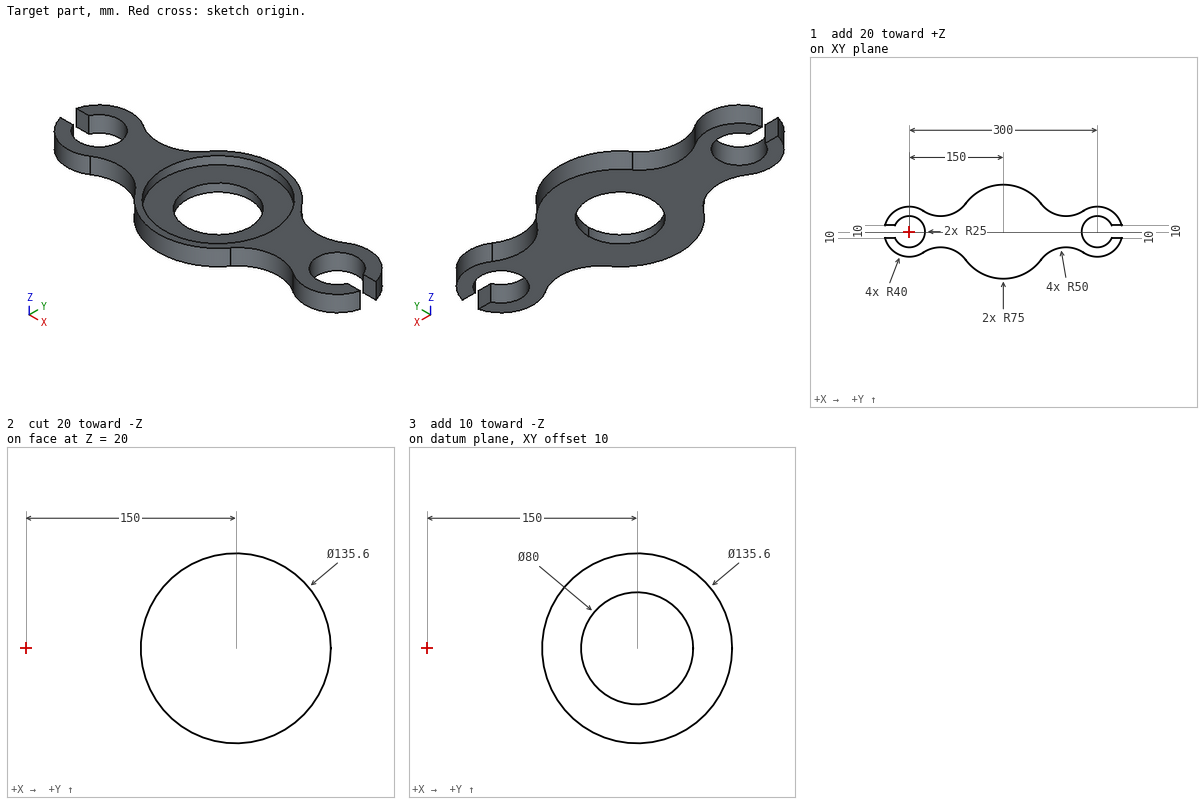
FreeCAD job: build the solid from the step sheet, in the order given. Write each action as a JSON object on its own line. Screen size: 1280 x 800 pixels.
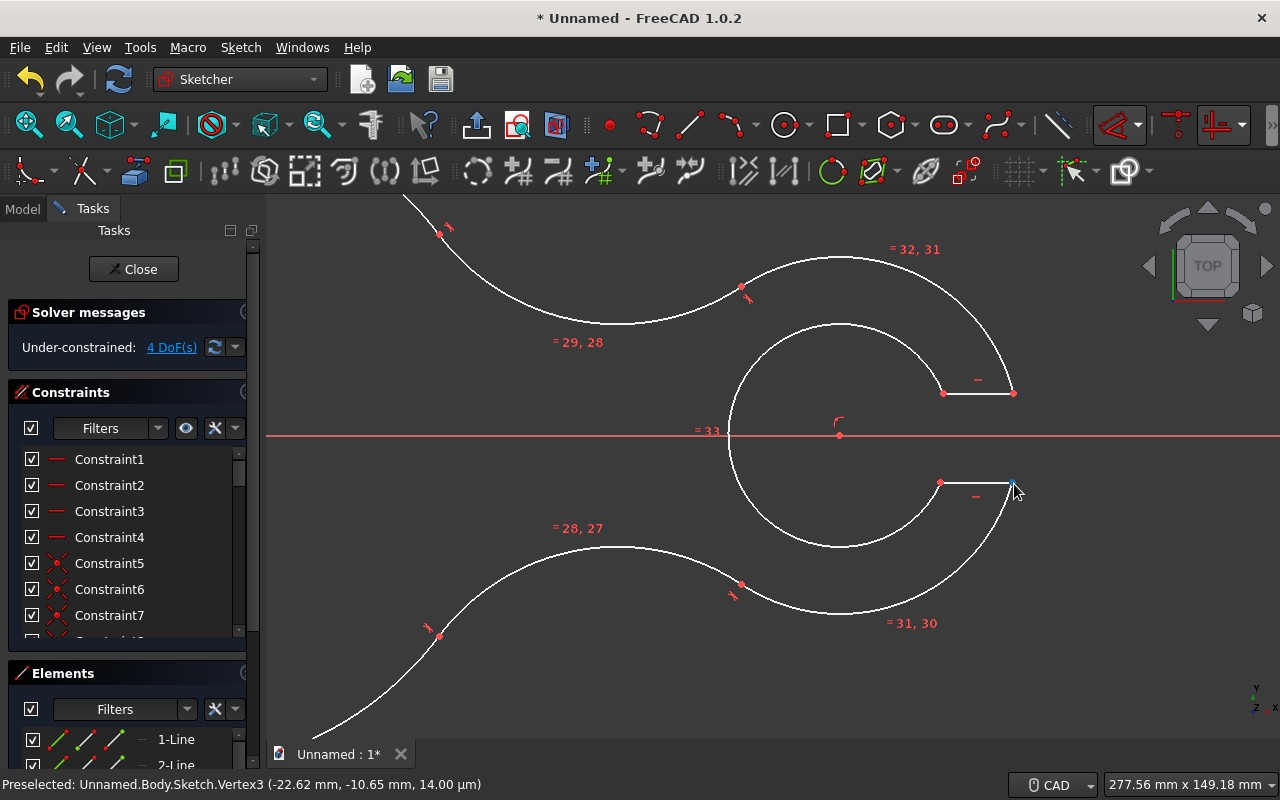
{"action": "left_click", "coordinate": [1012, 483]}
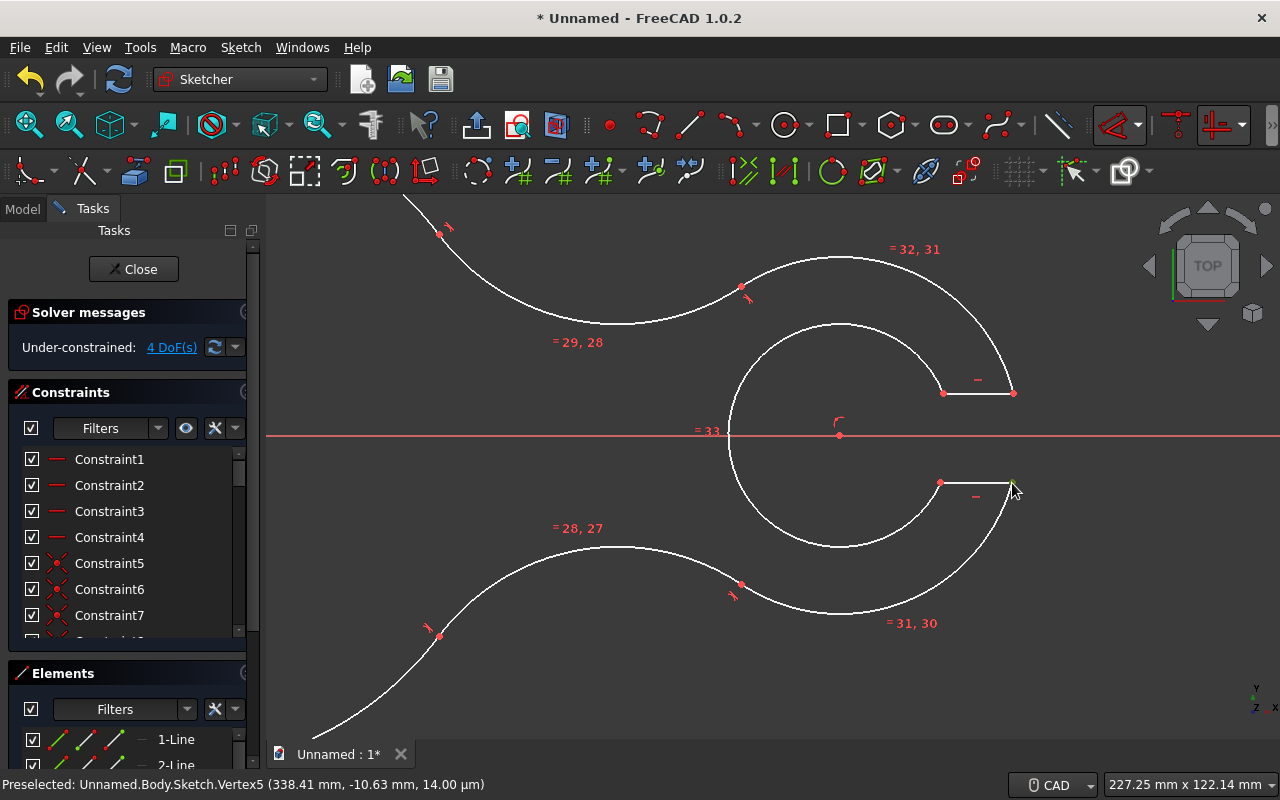
{"action": "left_click", "coordinate": [1140, 126]}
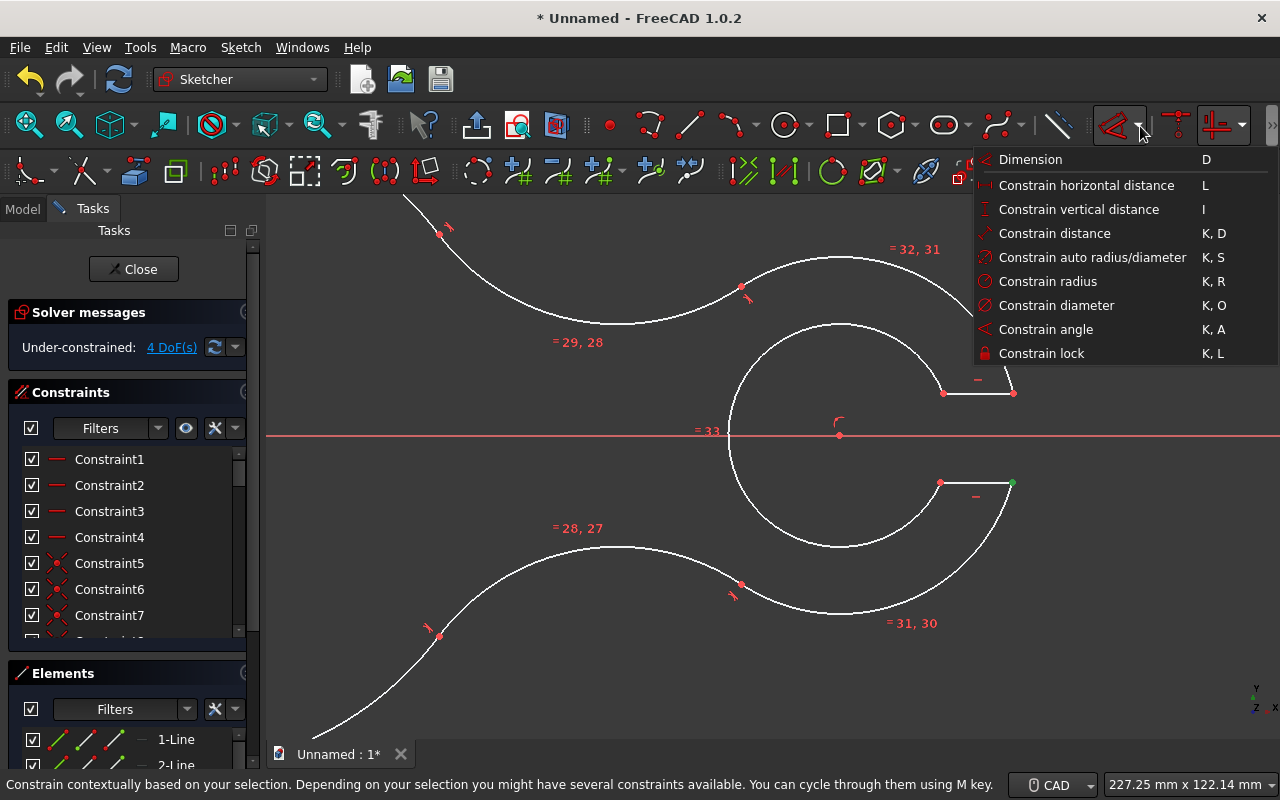
{"action": "left_click", "coordinate": [1126, 209]}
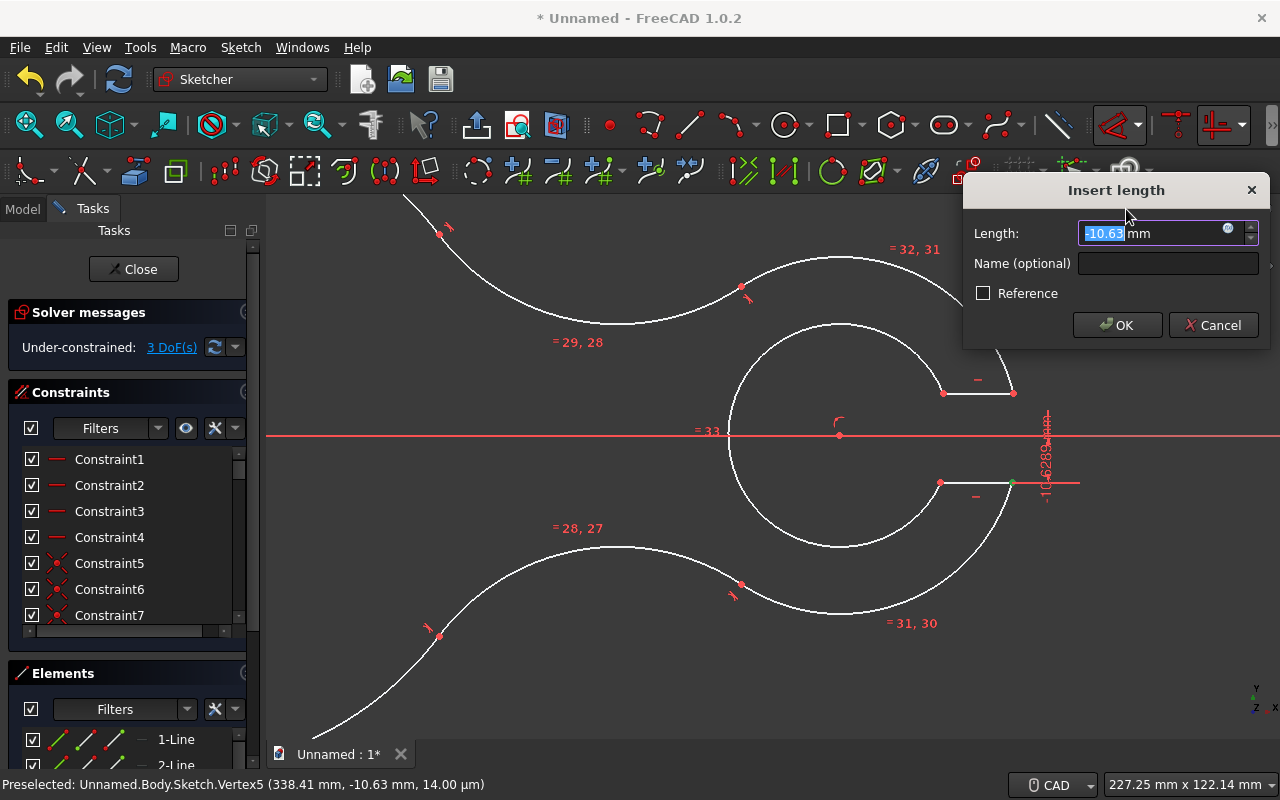
{"action": "type", "text": "-10"}
{"action": "key", "text": "Return"}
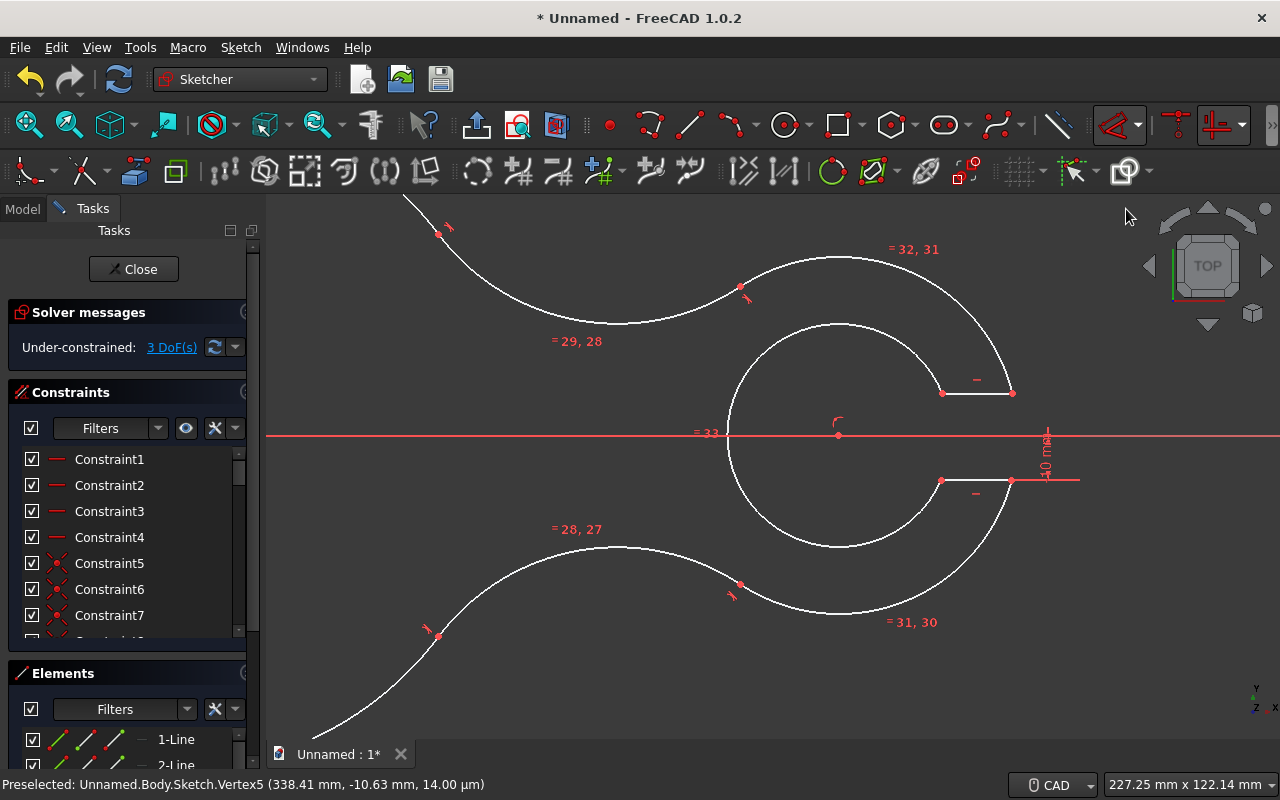
{"action": "left_click", "coordinate": [942, 394]}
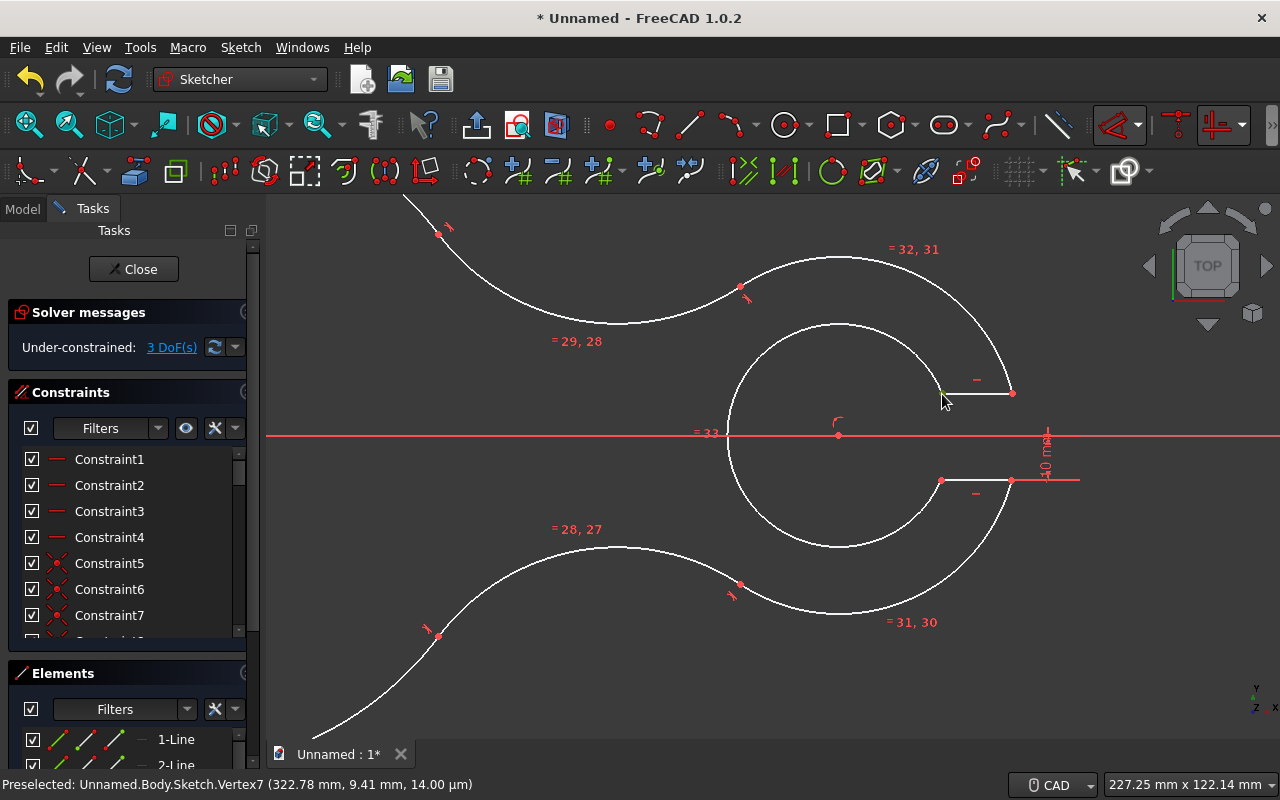
{"action": "left_click", "coordinate": [1140, 126]}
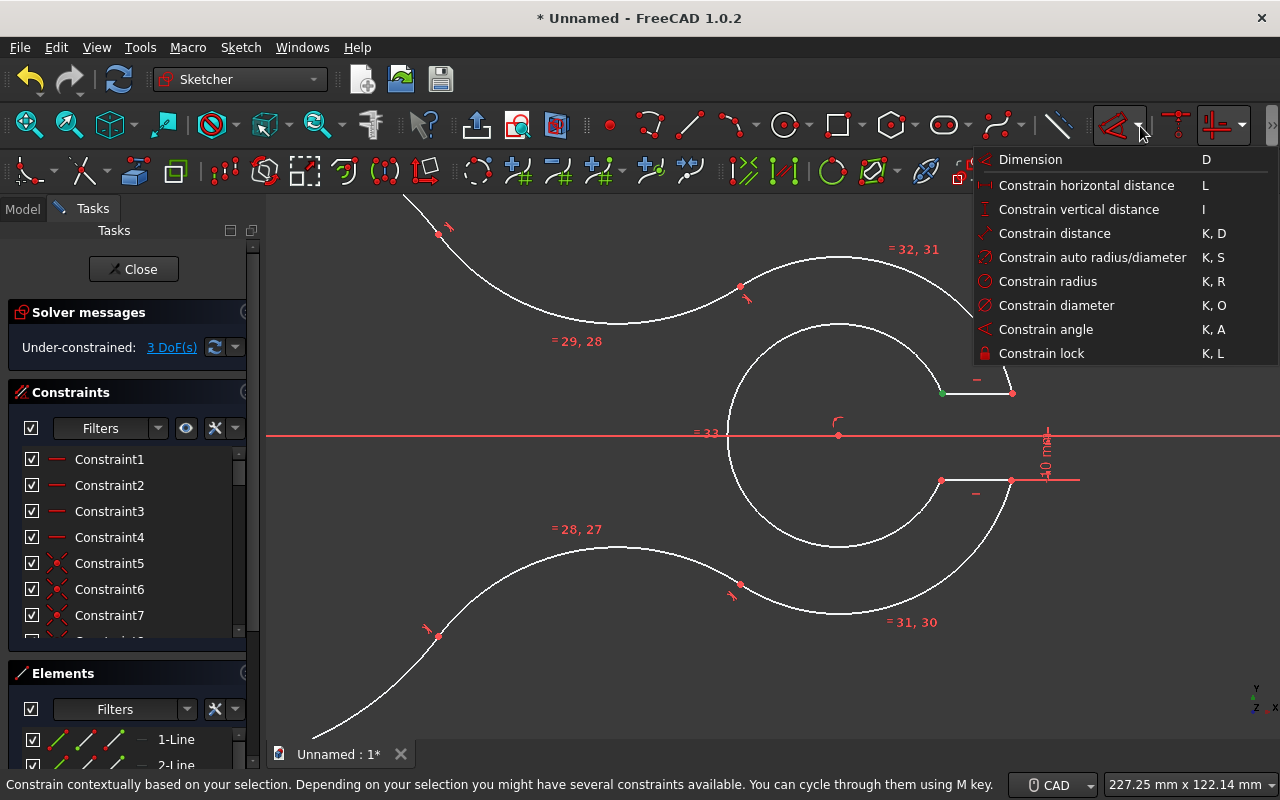
{"action": "left_click", "coordinate": [1126, 209]}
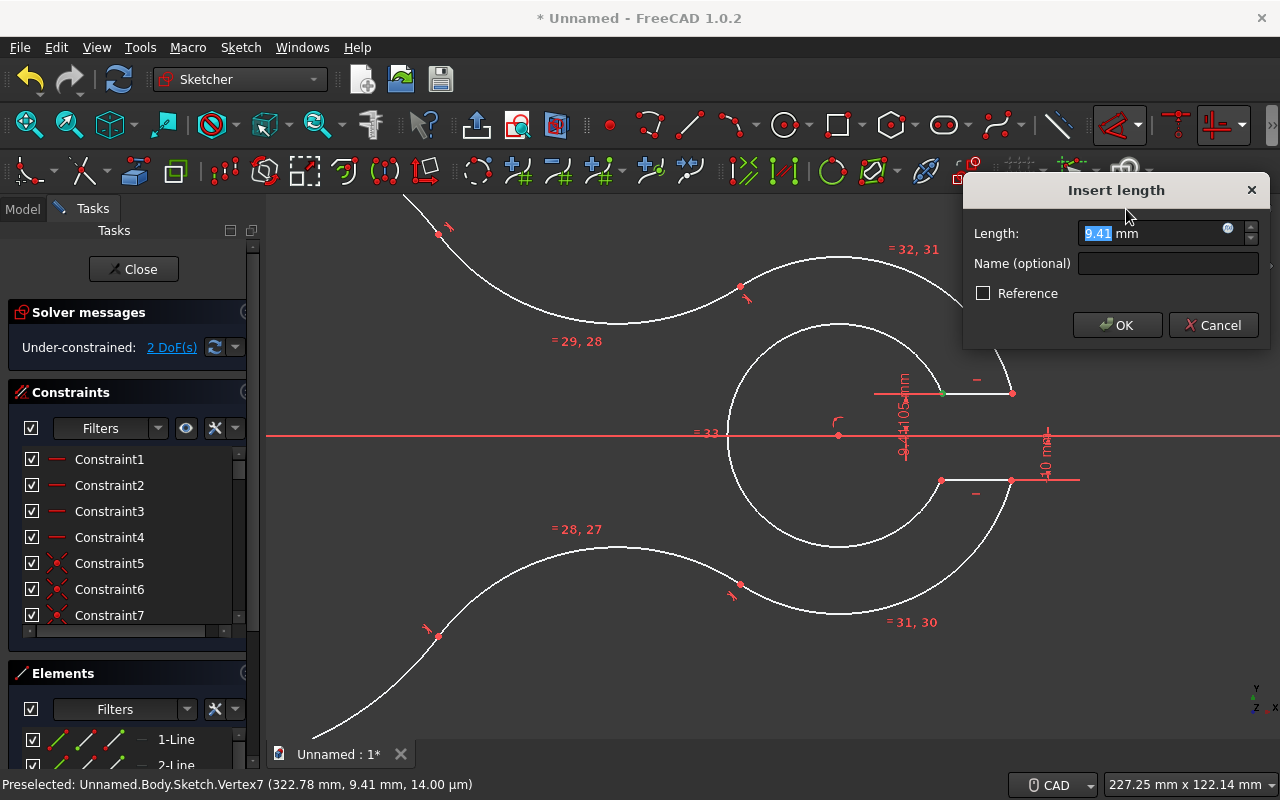
{"action": "type", "text": "10"}
{"action": "key", "text": "Return"}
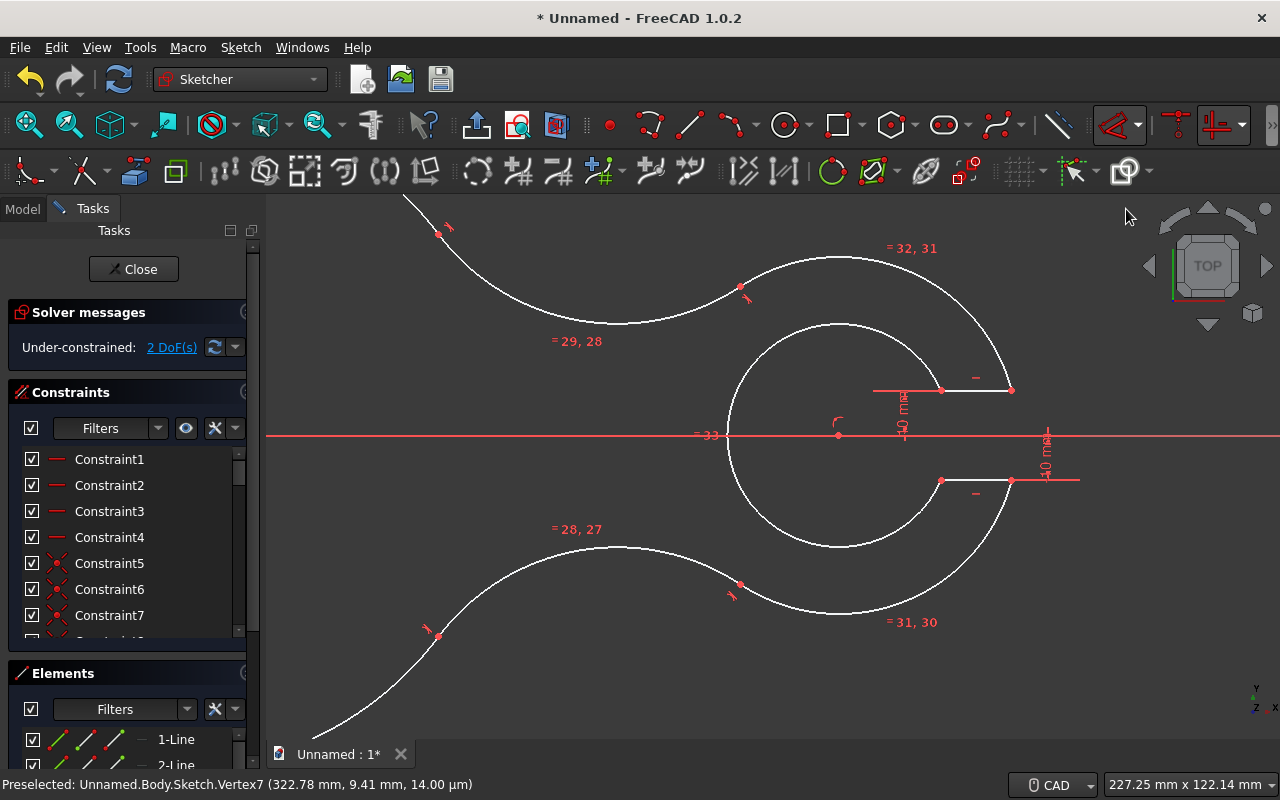
{"action": "scroll", "coordinate": [1015, 485], "scroll_direction": "down", "scroll_amount": 5}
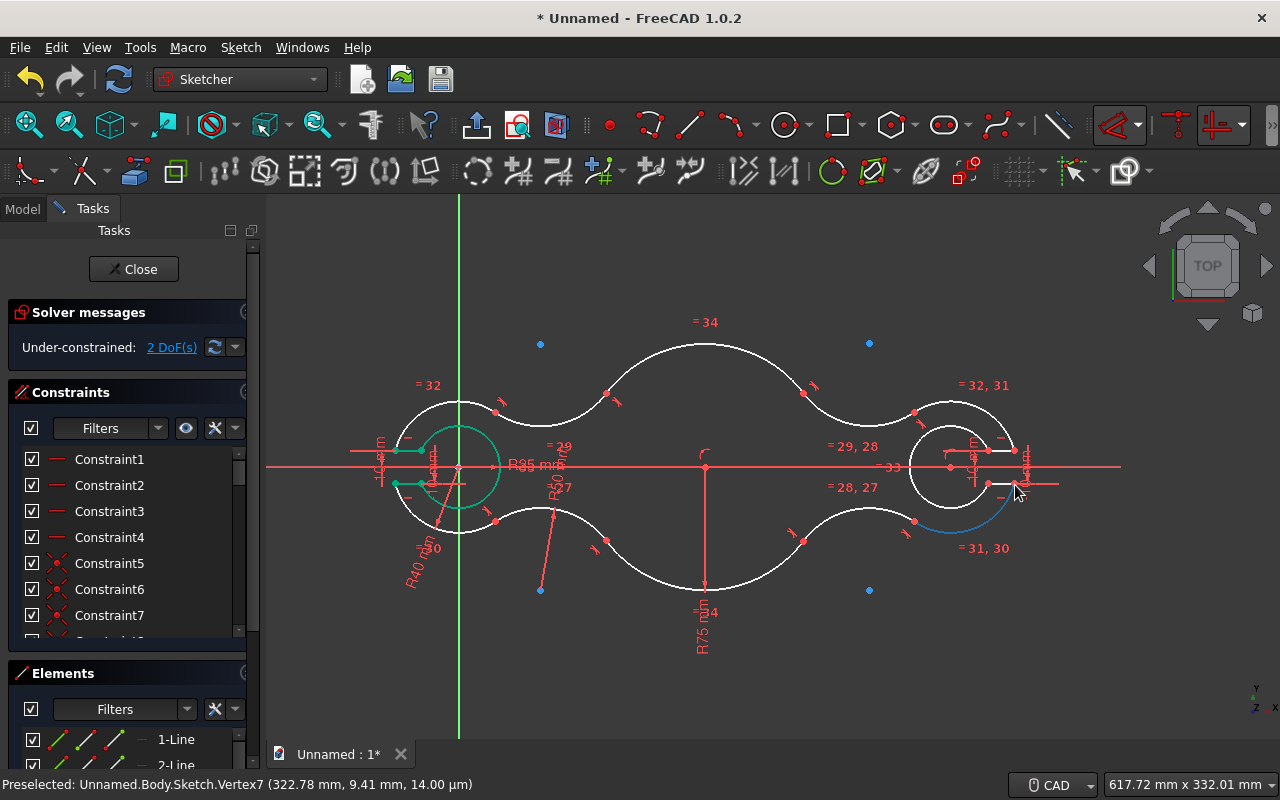
{"action": "left_click", "coordinate": [705, 467]}